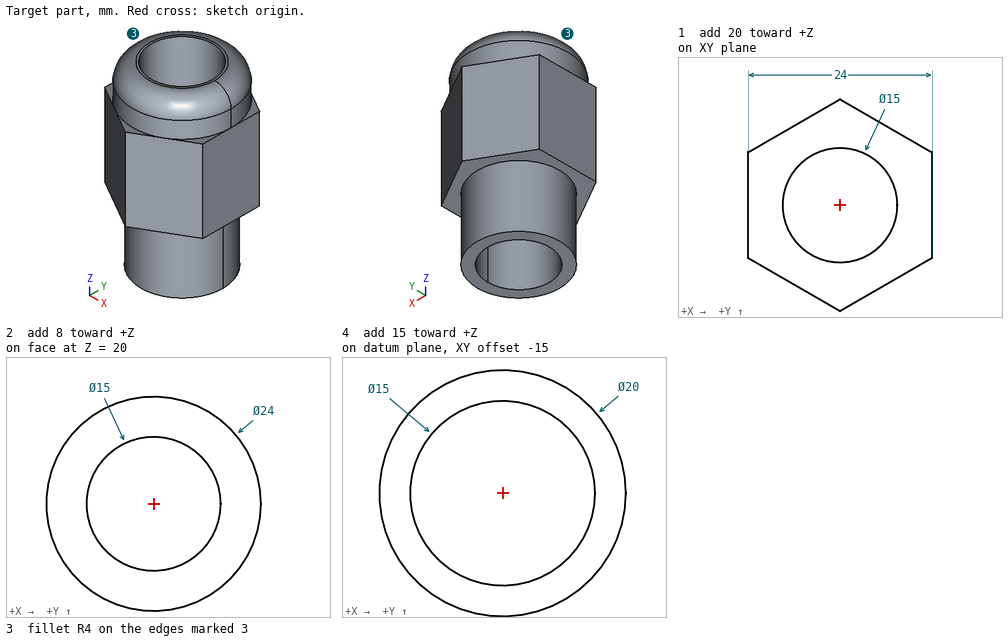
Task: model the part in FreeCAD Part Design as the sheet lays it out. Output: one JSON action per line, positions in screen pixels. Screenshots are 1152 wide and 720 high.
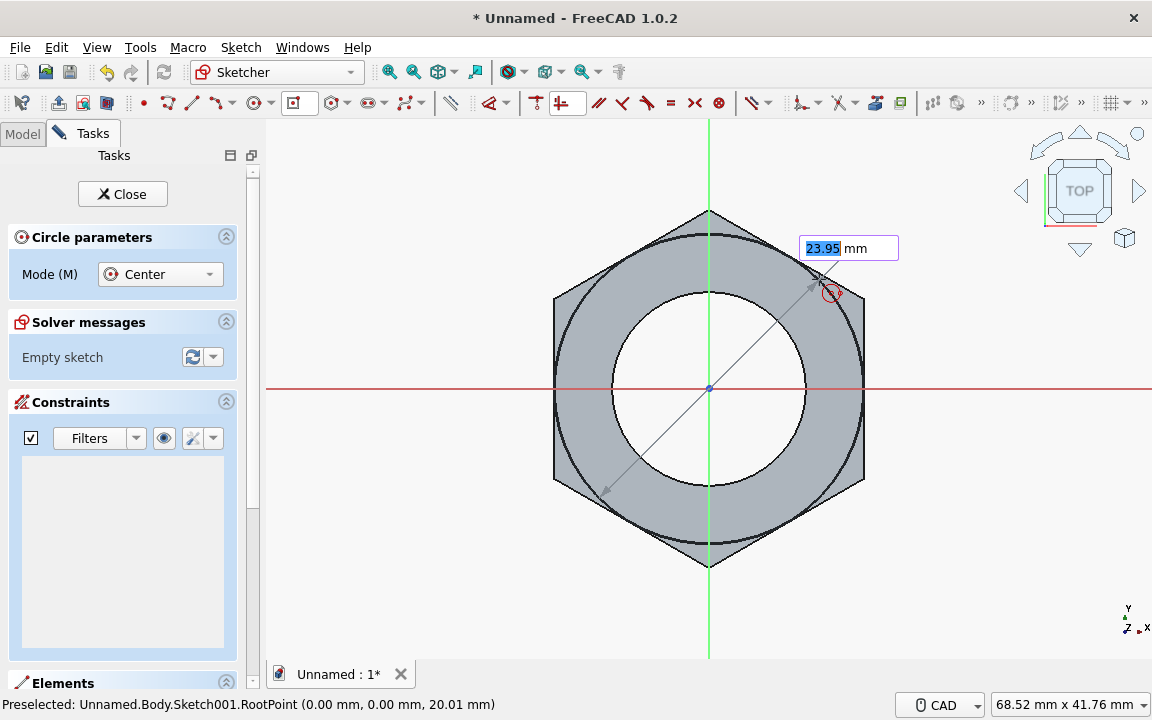
{"action": "type", "text": "24"}
{"action": "key", "text": "Return"}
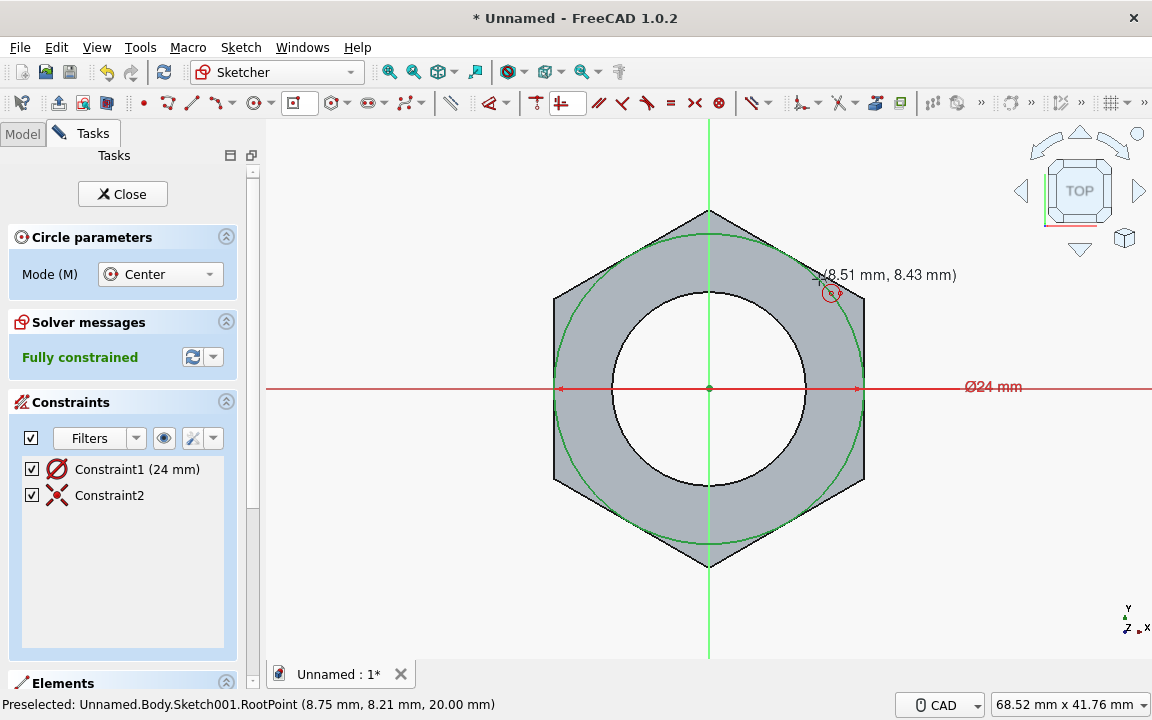
{"action": "left_click", "coordinate": [709, 389]}
{"action": "mouse_move", "coordinate": [778, 320]}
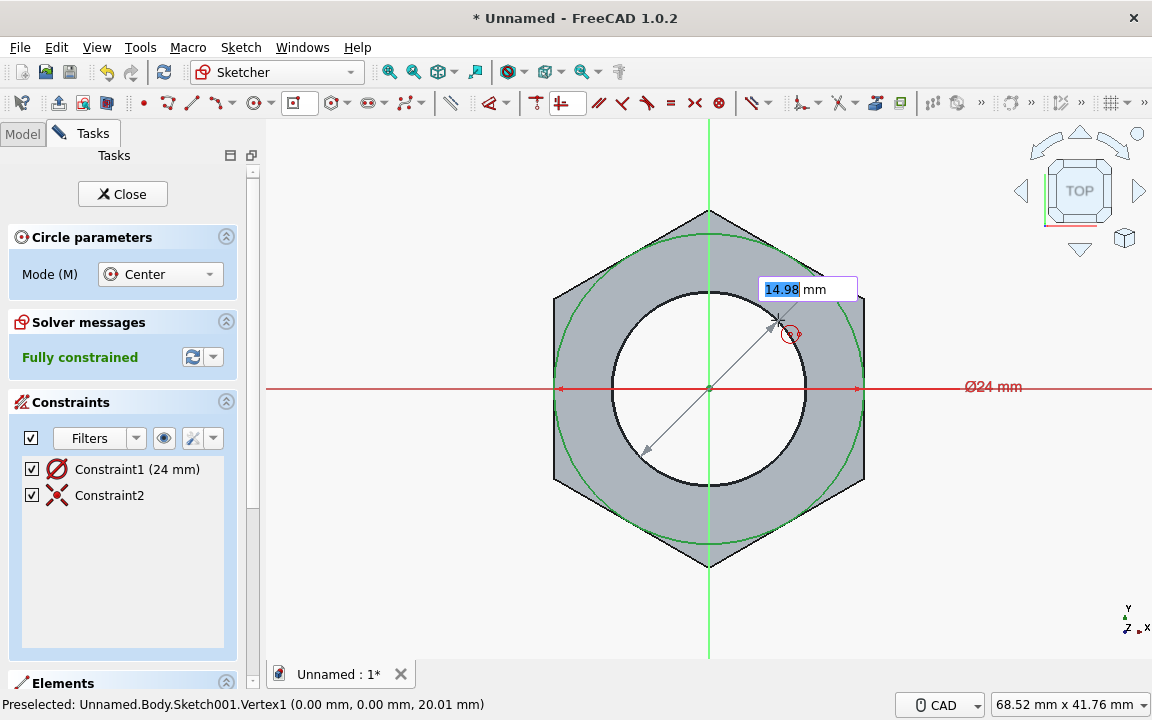
{"action": "type", "text": "15"}
{"action": "key", "text": "Return"}
{"action": "key", "text": "Escape"}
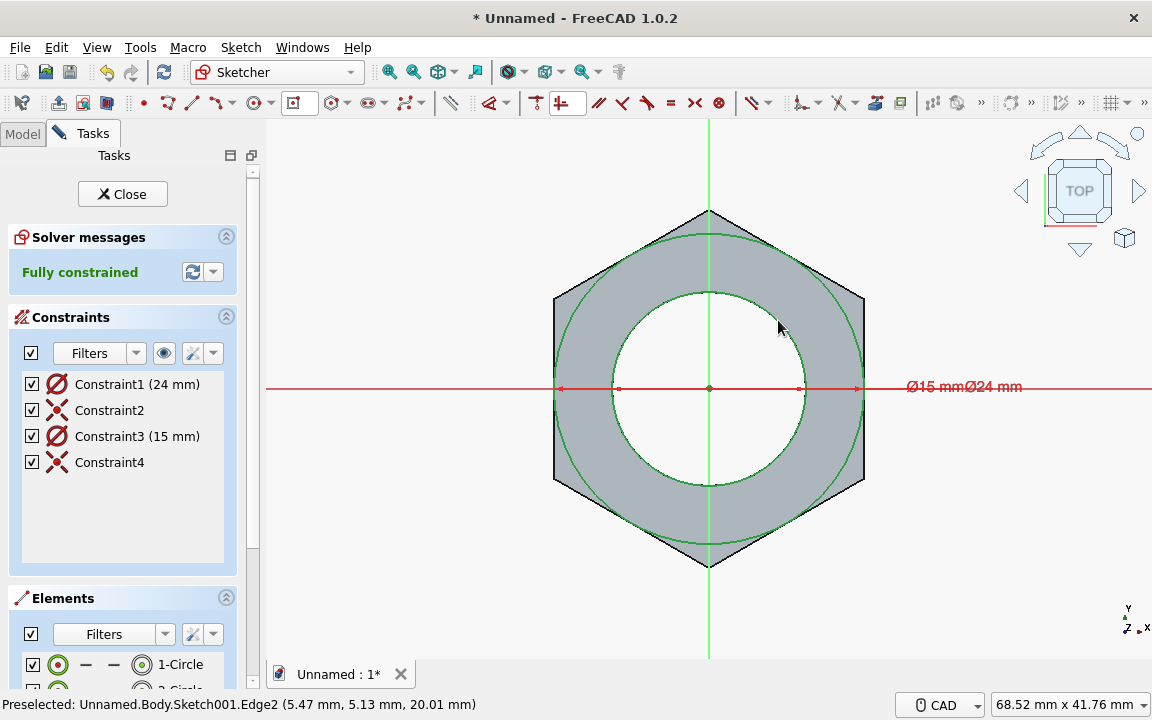
{"action": "left_click", "coordinate": [123, 194]}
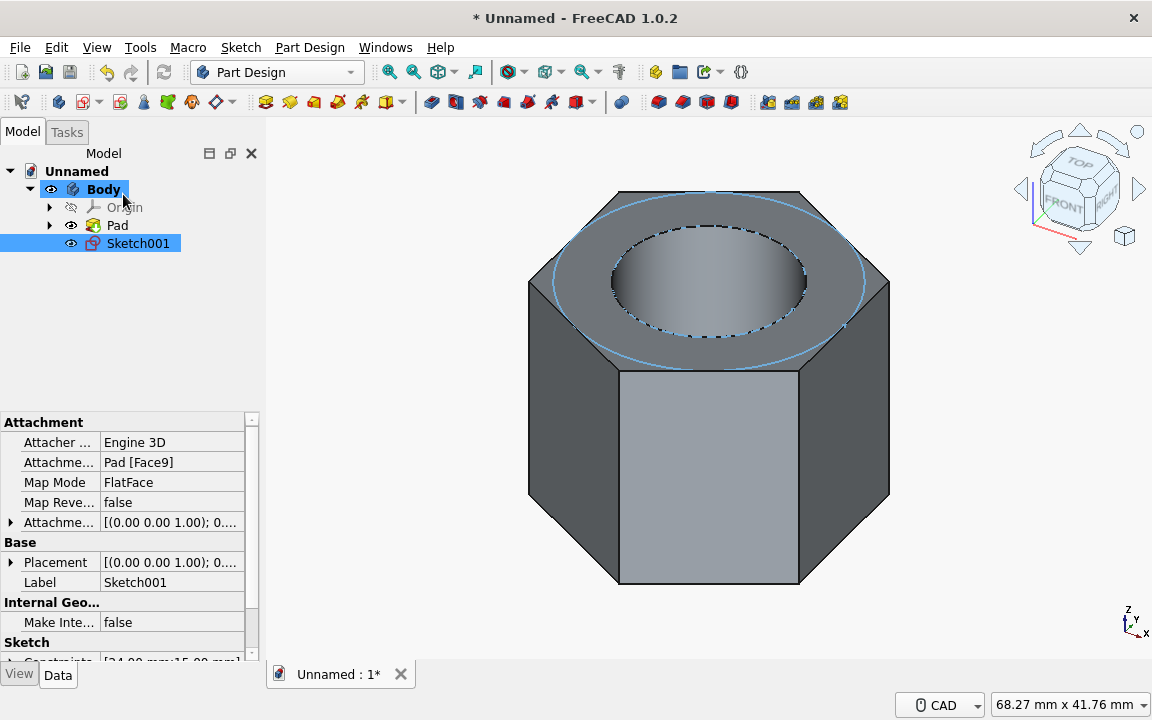
{"action": "left_click", "coordinate": [266, 102]}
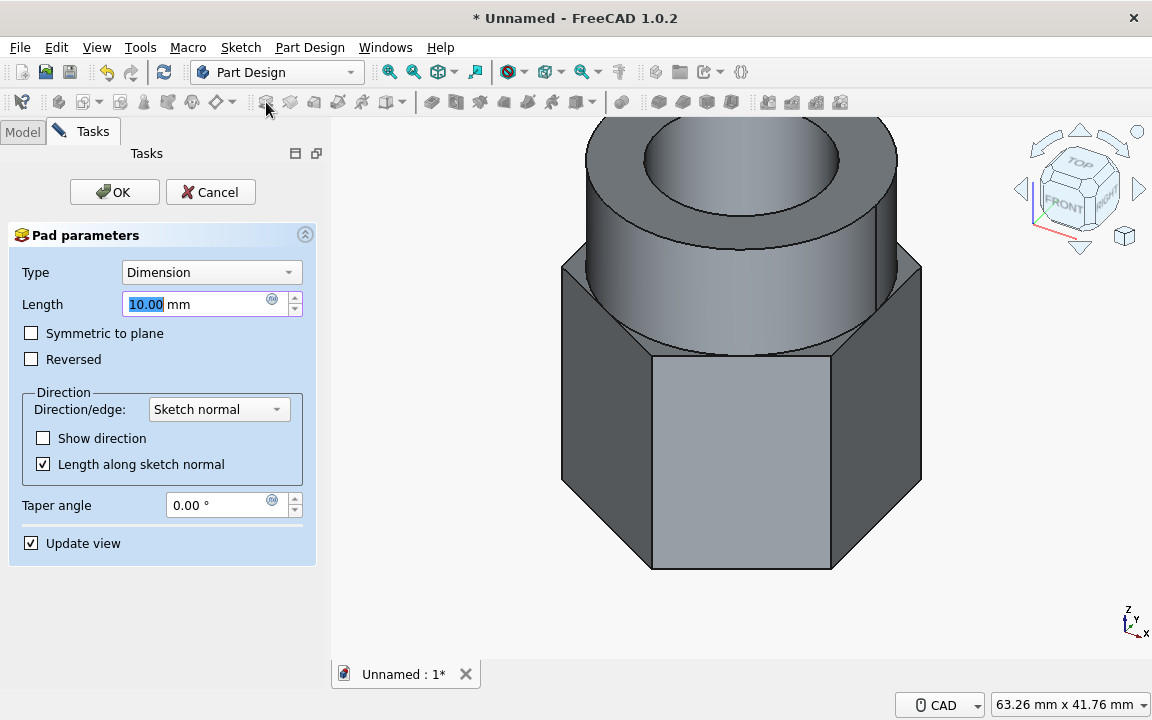
{"action": "type", "text": "8"}
{"action": "key", "text": "Tab"}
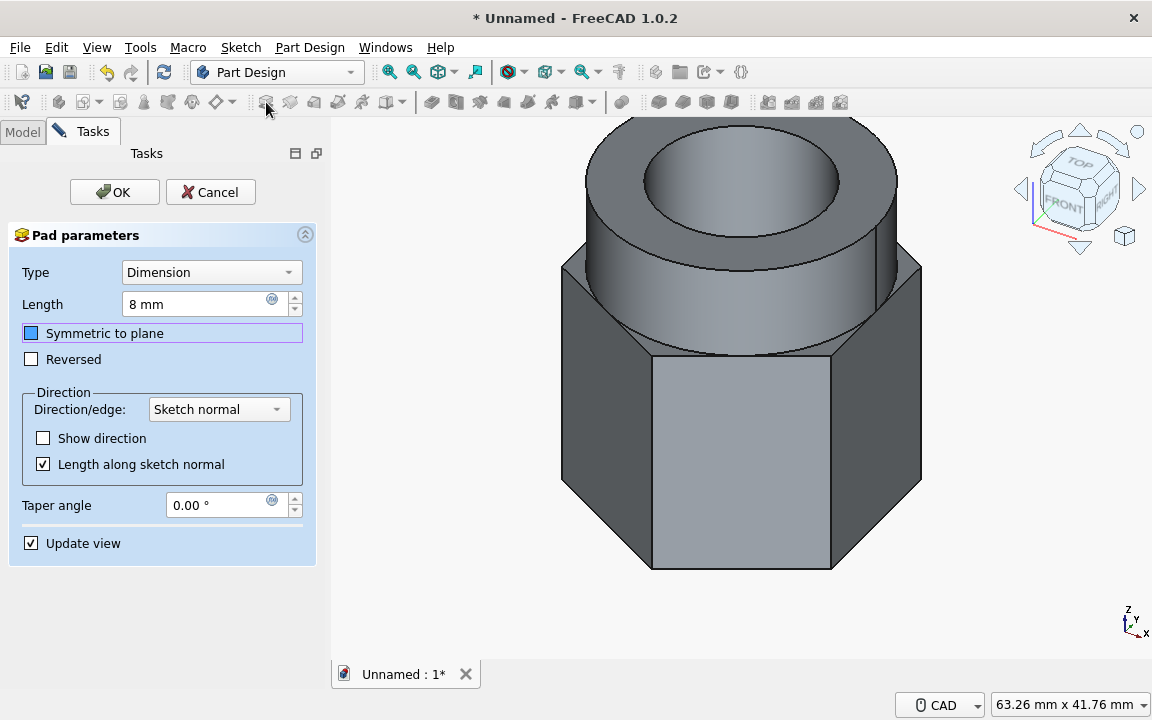
{"action": "left_click", "coordinate": [115, 192]}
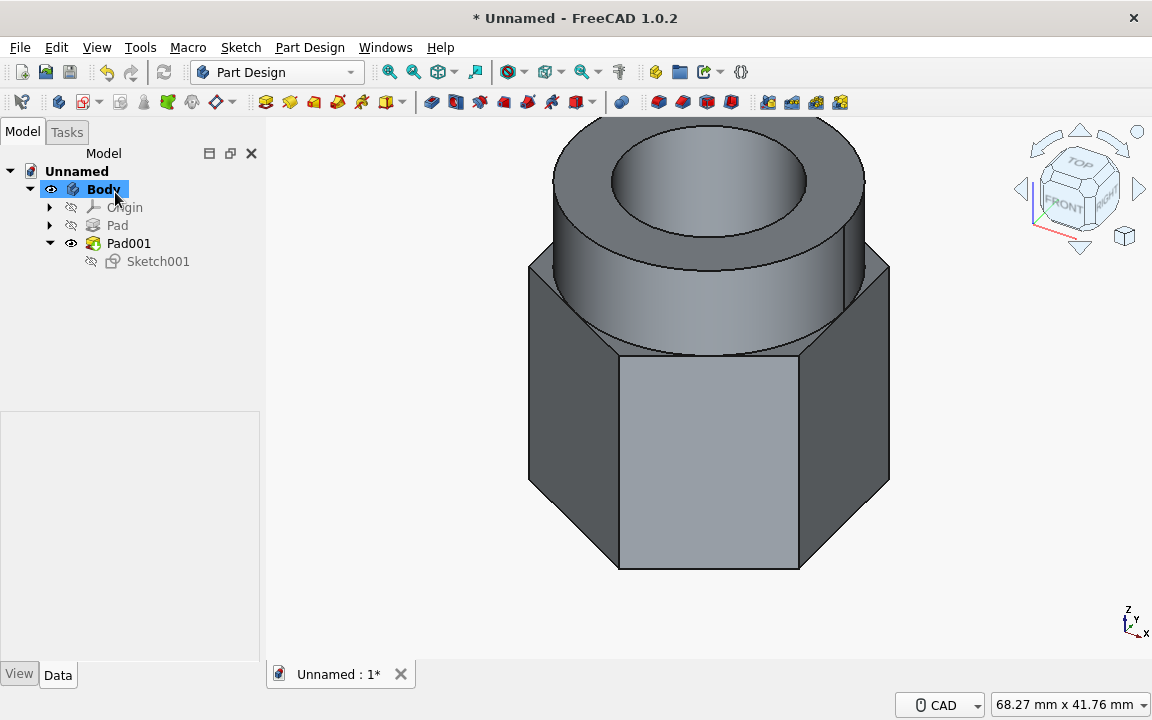
{"action": "left_click", "coordinate": [390, 72]}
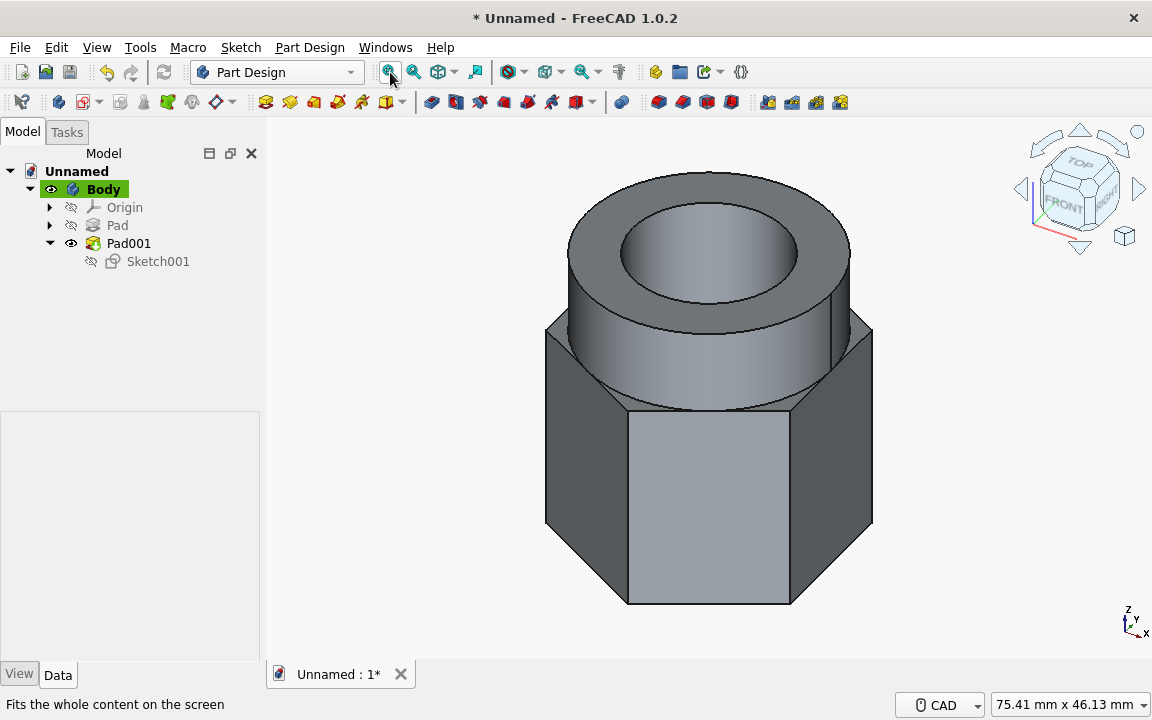
{"action": "left_click", "coordinate": [569, 261]}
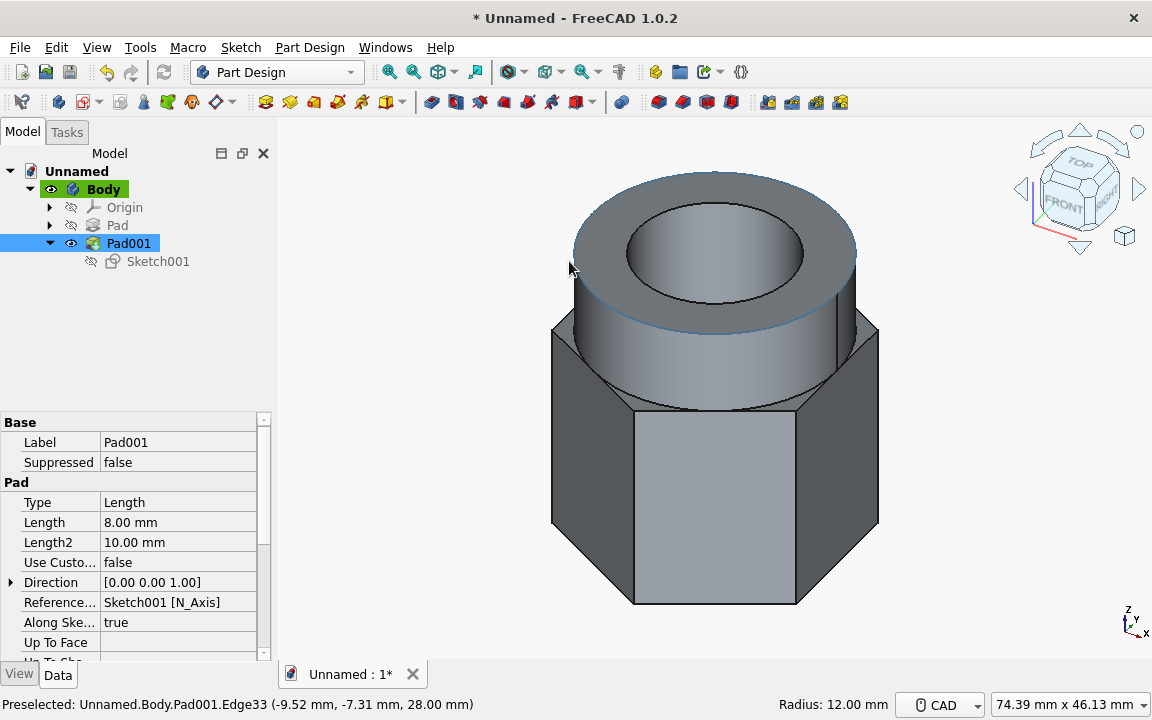
{"action": "left_click", "coordinate": [660, 102]}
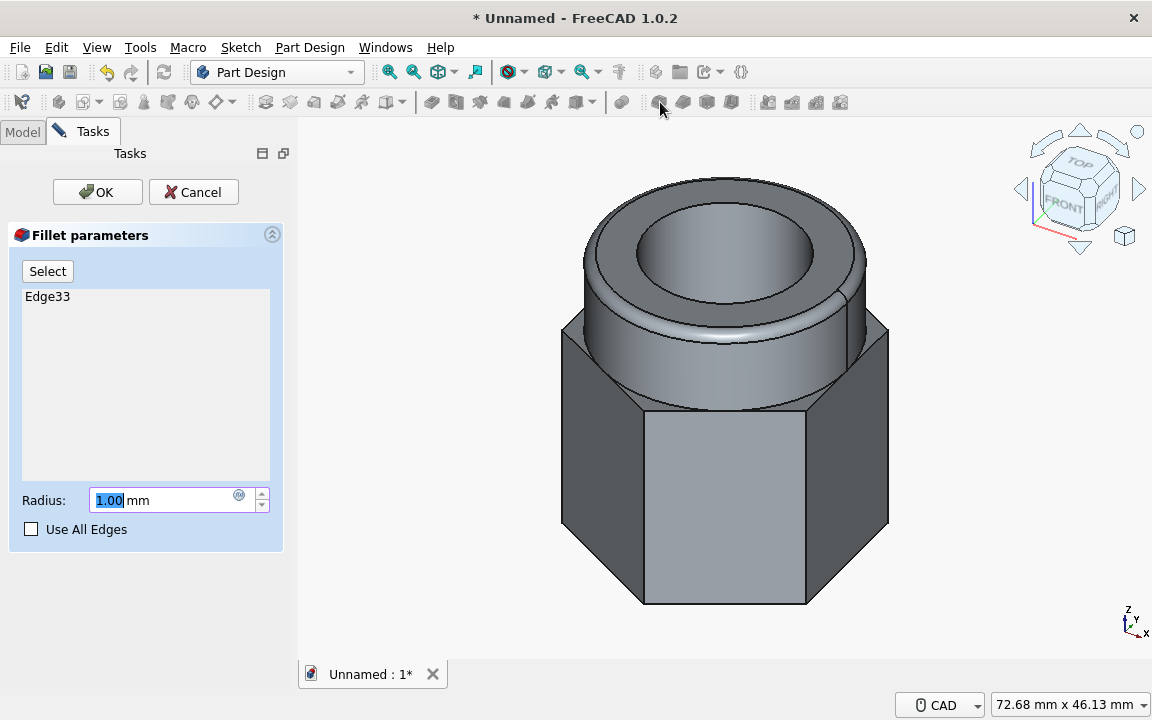
{"action": "type", "text": "4"}
{"action": "key", "text": "Tab"}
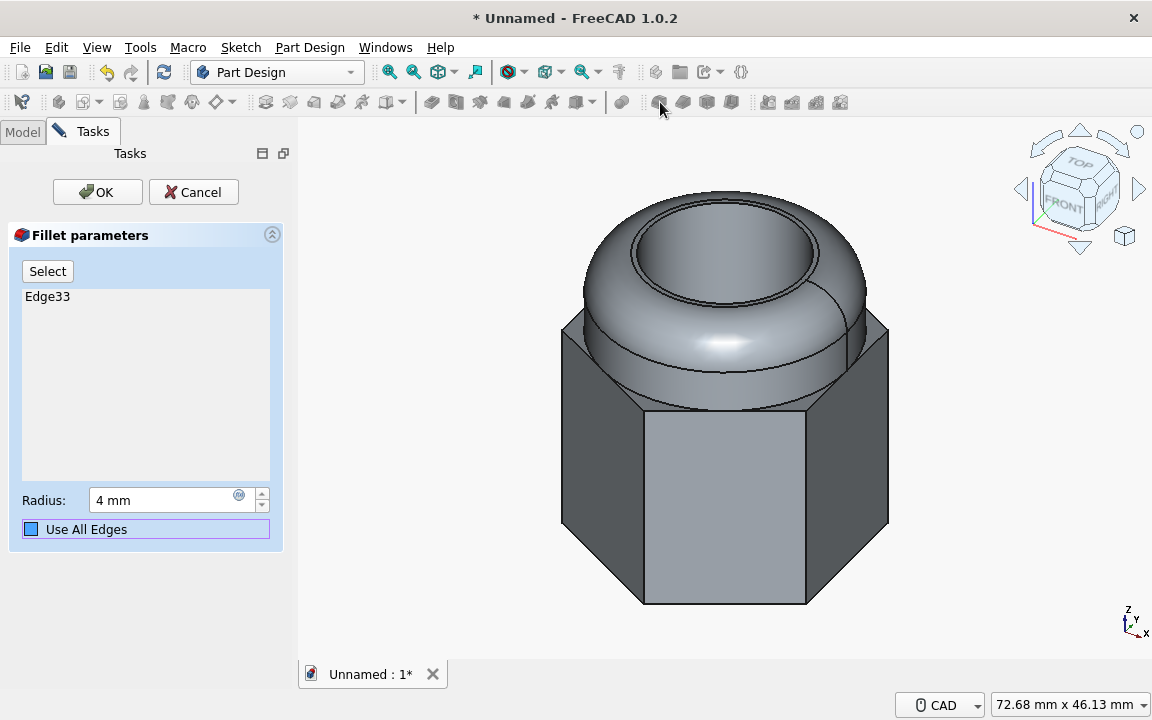
{"action": "left_click", "coordinate": [98, 192]}